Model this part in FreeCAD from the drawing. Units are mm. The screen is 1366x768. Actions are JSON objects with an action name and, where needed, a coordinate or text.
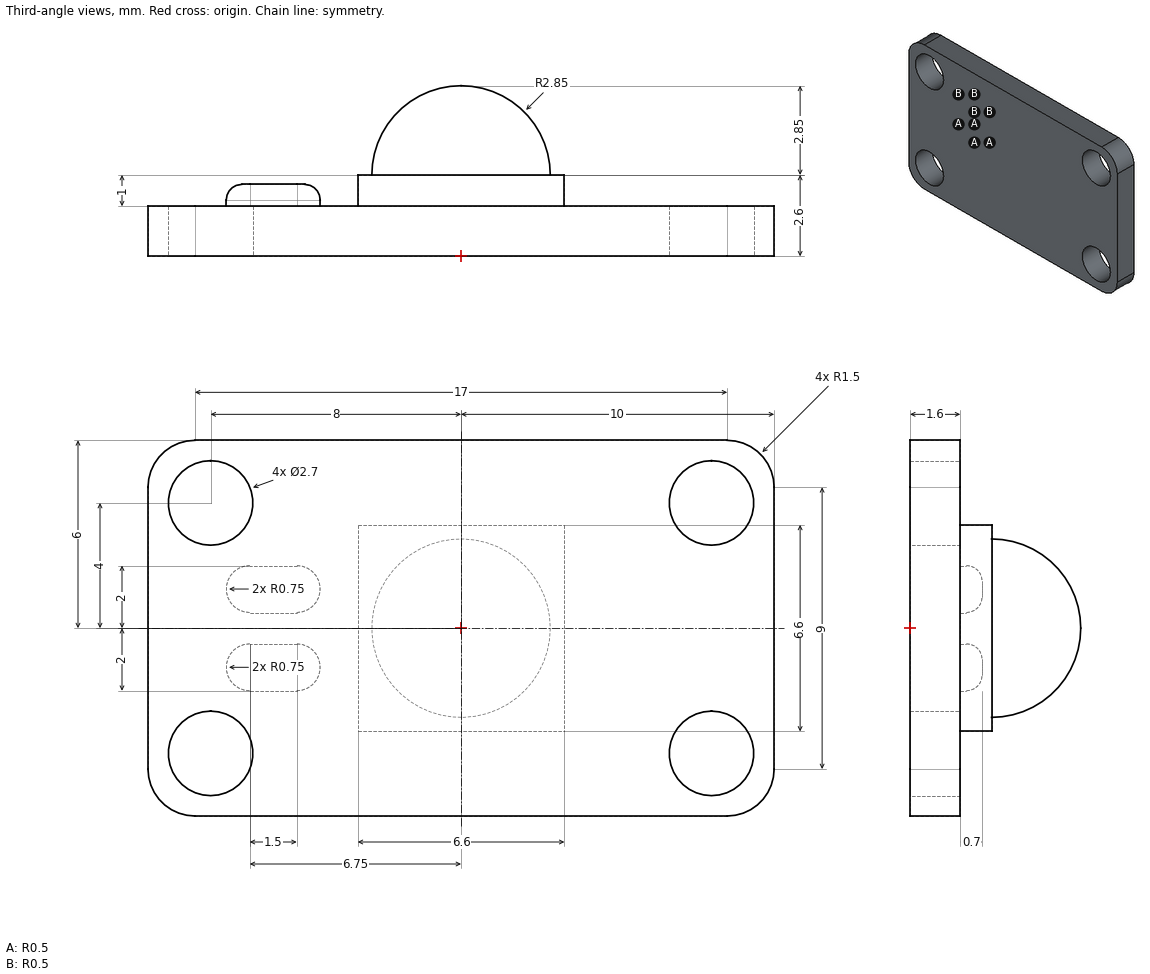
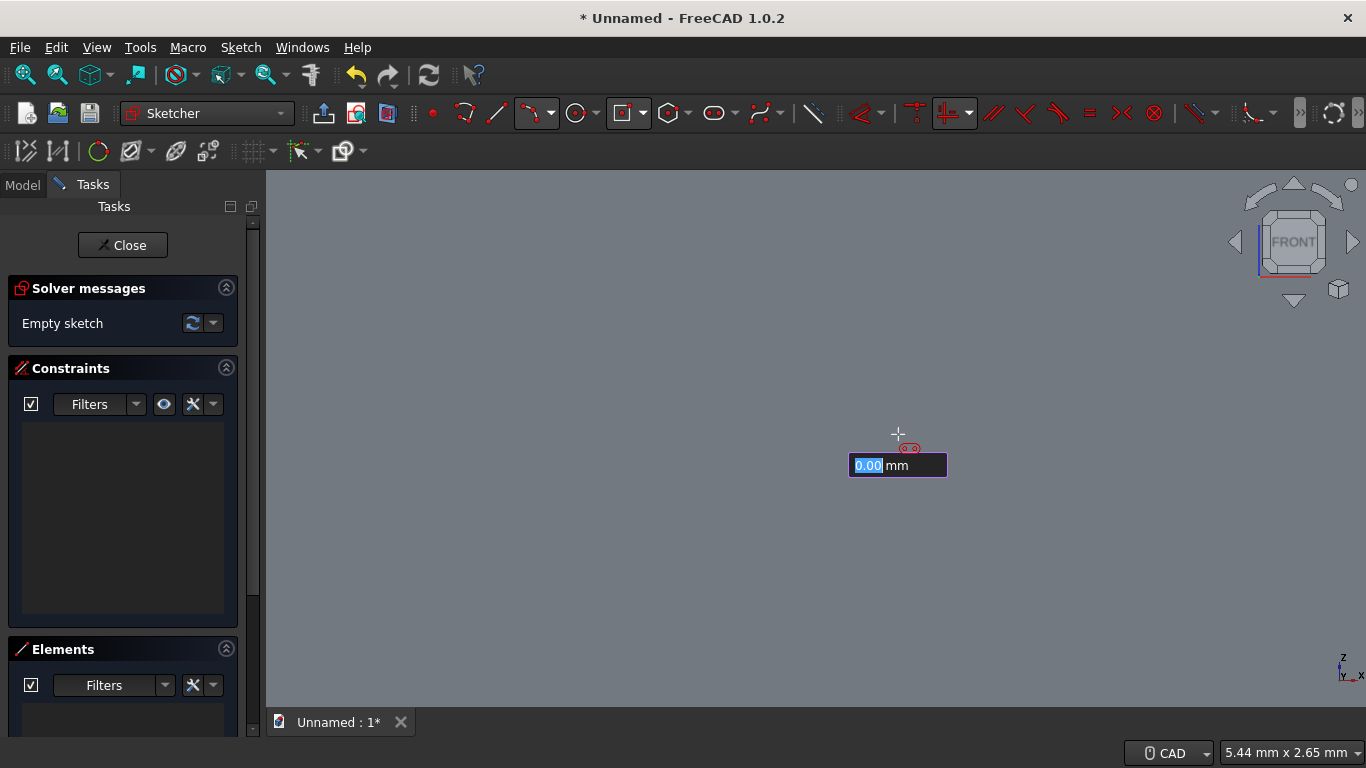
{"action": "left_click", "coordinate": [747, 586]}
{"action": "key", "text": "Escape"}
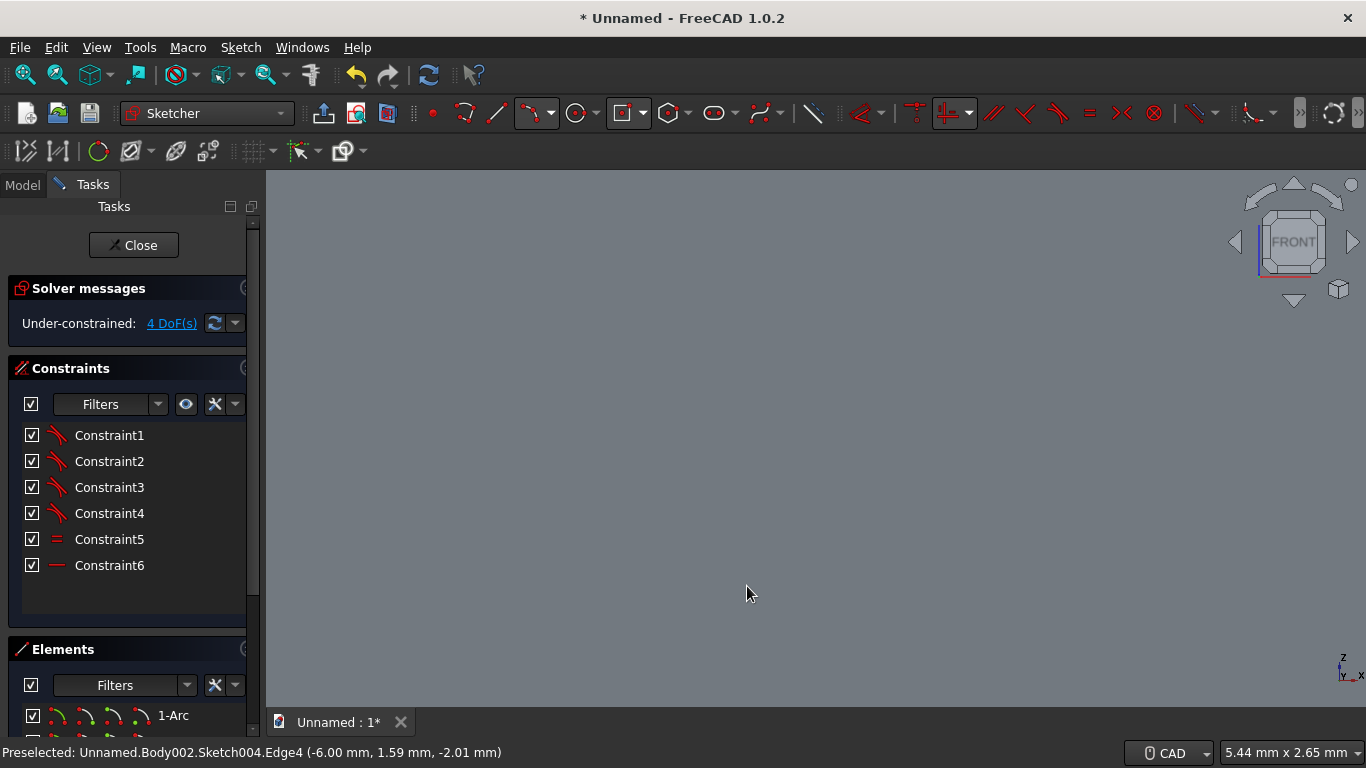
{"action": "left_click", "coordinate": [860, 114]}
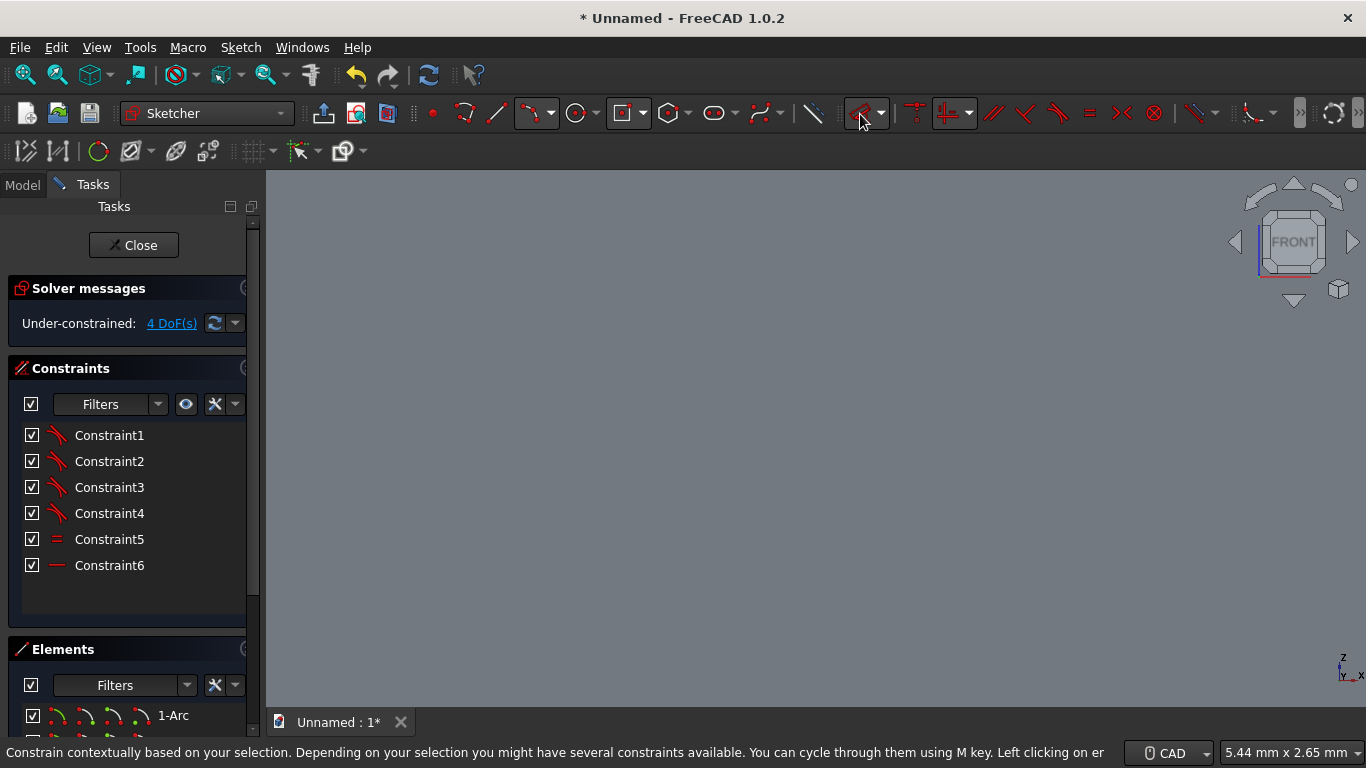
{"action": "left_click", "coordinate": [472, 346]}
{"action": "left_click", "coordinate": [446, 327]}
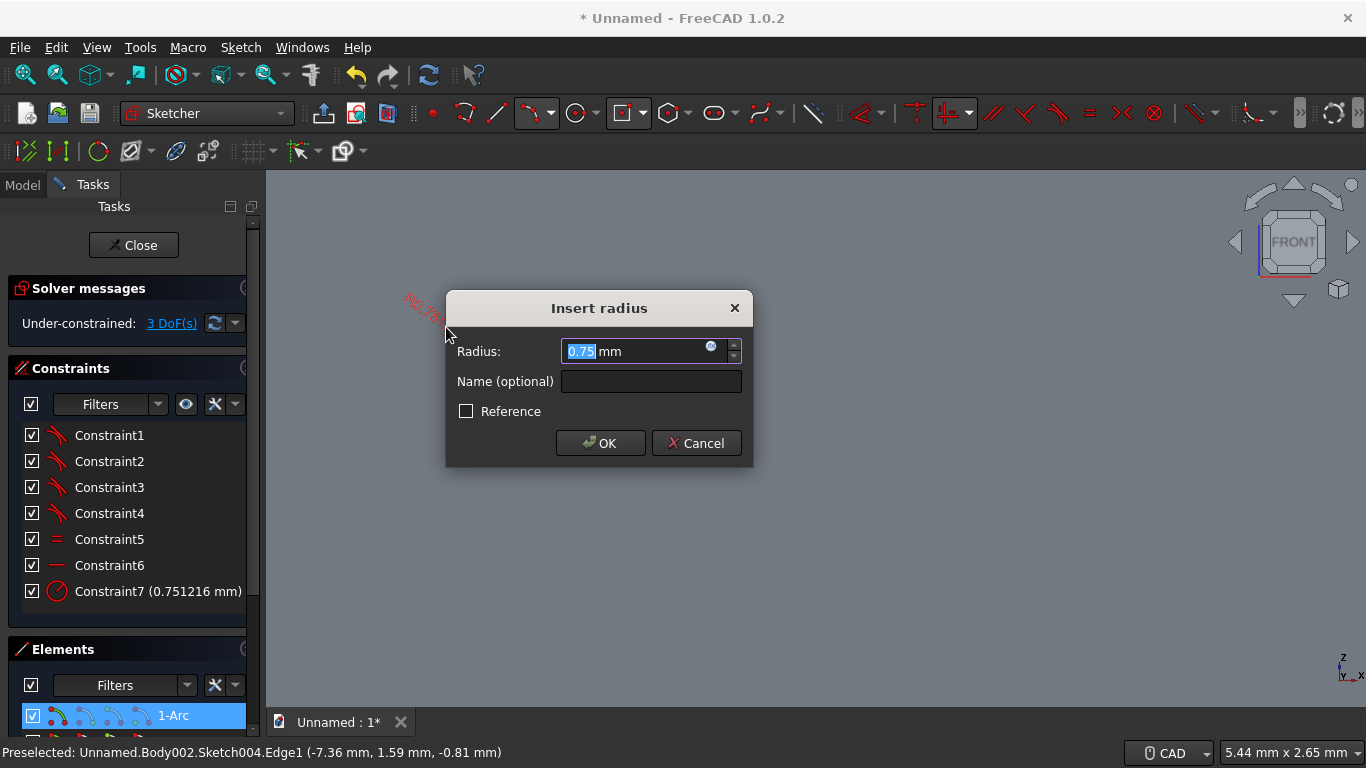
{"action": "type", "text": "0.75"}
{"action": "key", "text": "Return"}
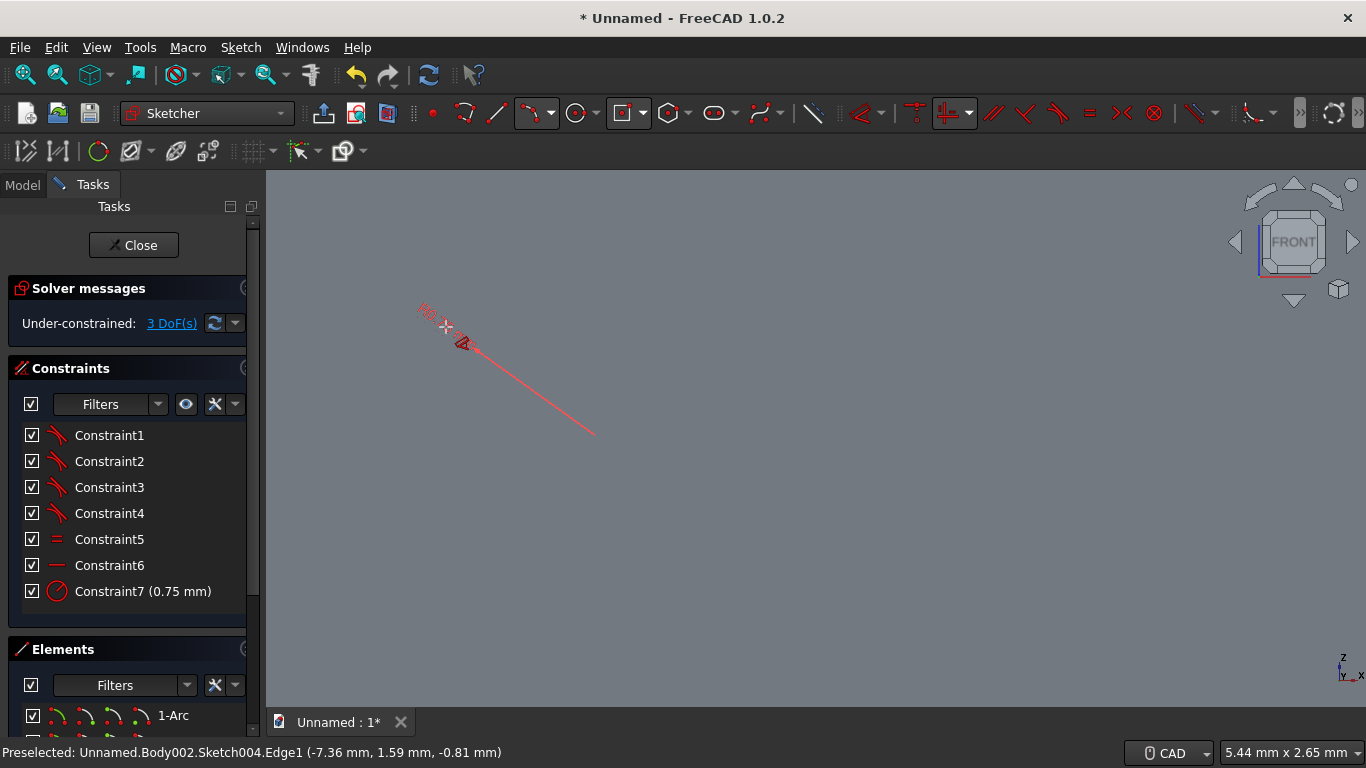
{"action": "left_click", "coordinate": [595, 587]}
{"action": "left_click", "coordinate": [561, 392]}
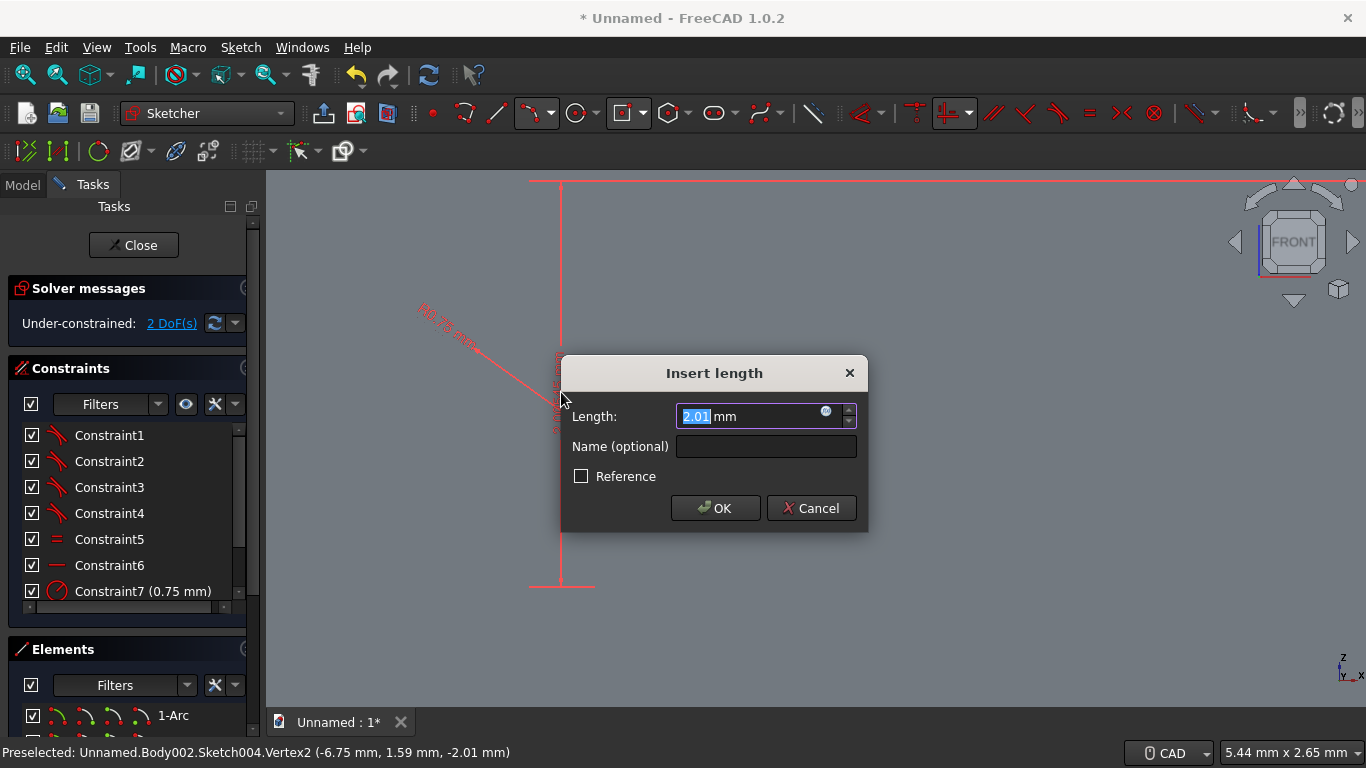
{"action": "type", "text": "2"}
{"action": "key", "text": "Return"}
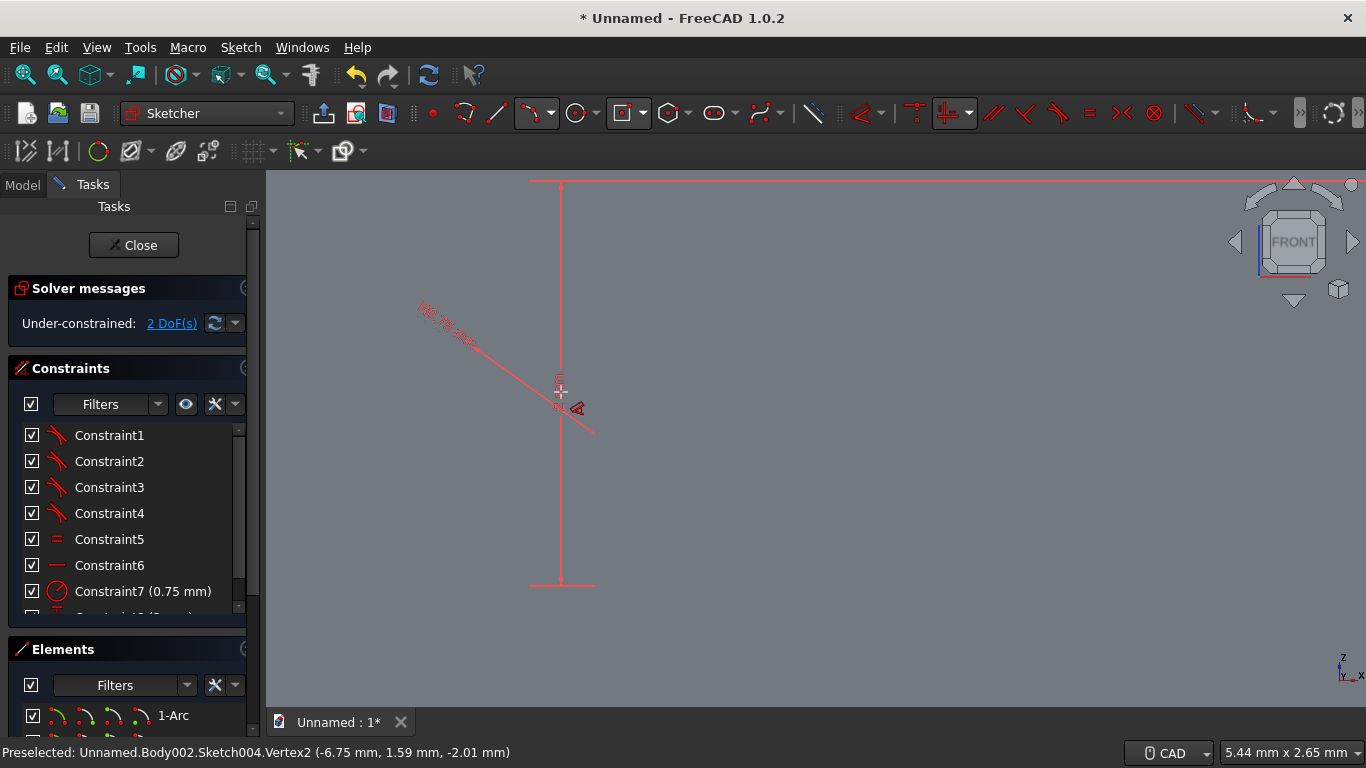
{"action": "left_click", "coordinate": [686, 282]}
{"action": "left_click", "coordinate": [746, 248]}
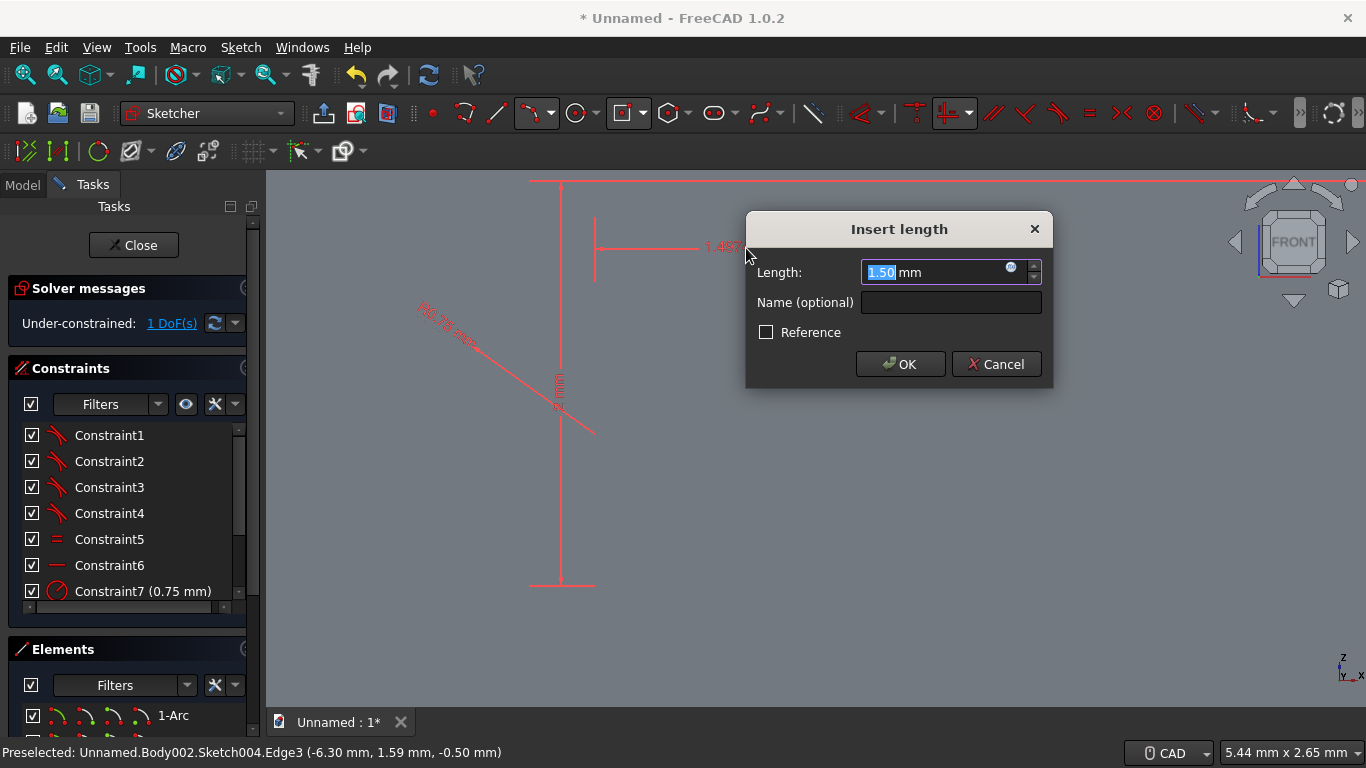
{"action": "type", "text": "1.5"}
{"action": "key", "text": "Return"}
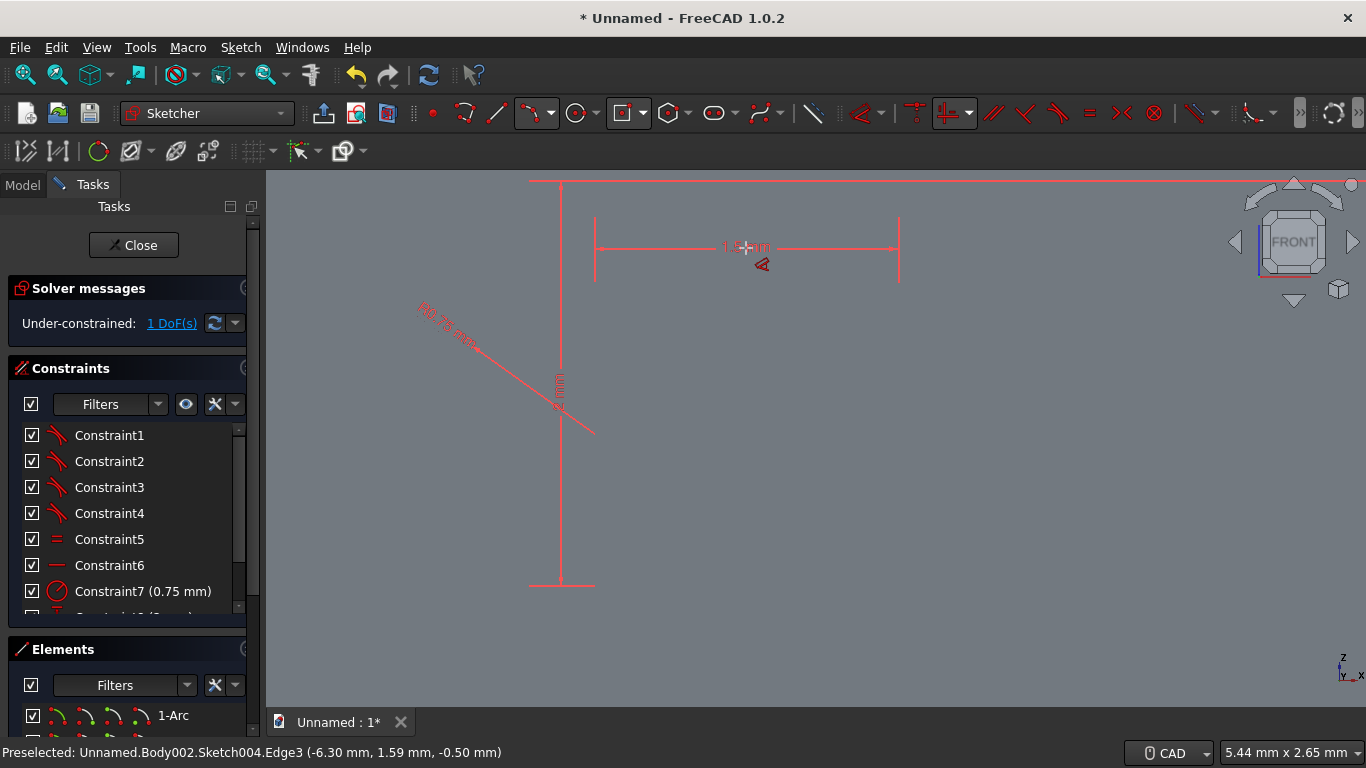
{"action": "left_click", "coordinate": [595, 282]}
{"action": "left_click", "coordinate": [898, 316]}